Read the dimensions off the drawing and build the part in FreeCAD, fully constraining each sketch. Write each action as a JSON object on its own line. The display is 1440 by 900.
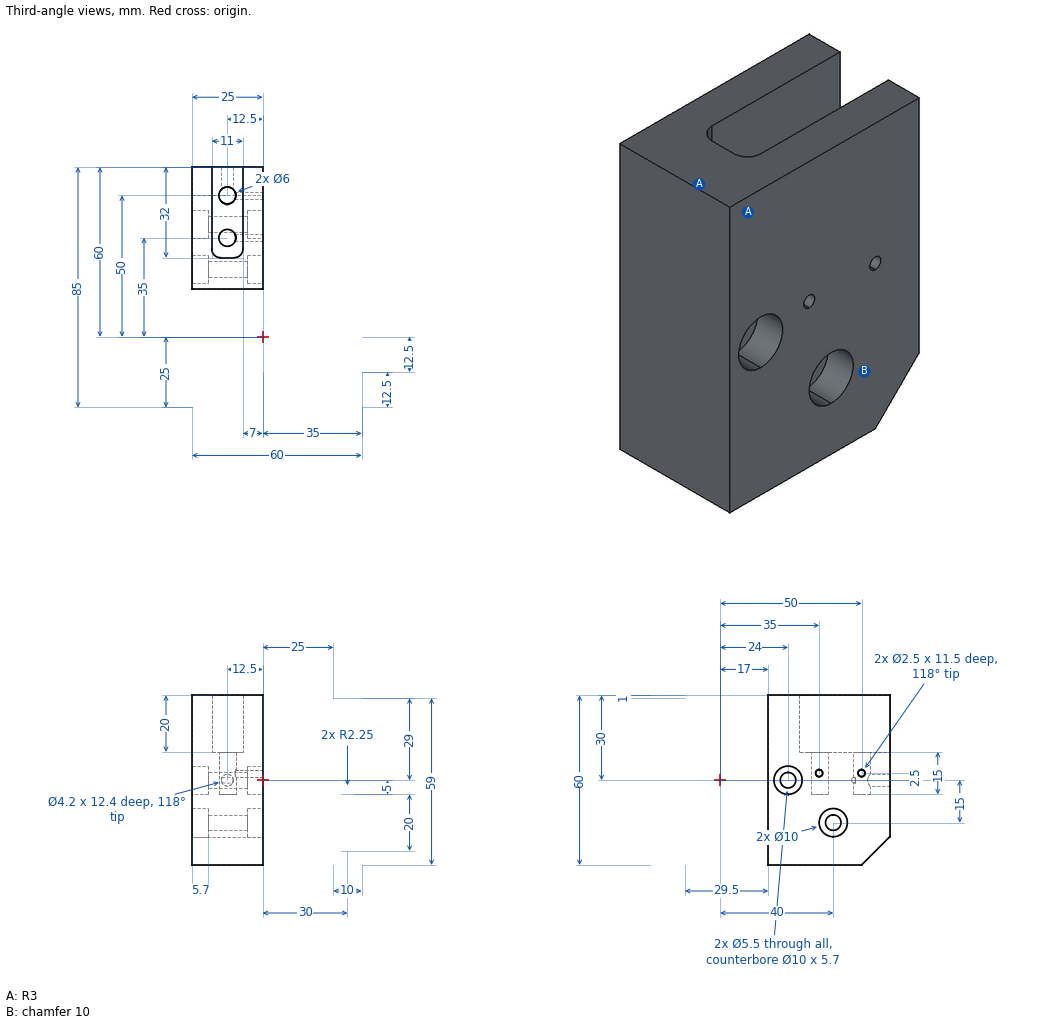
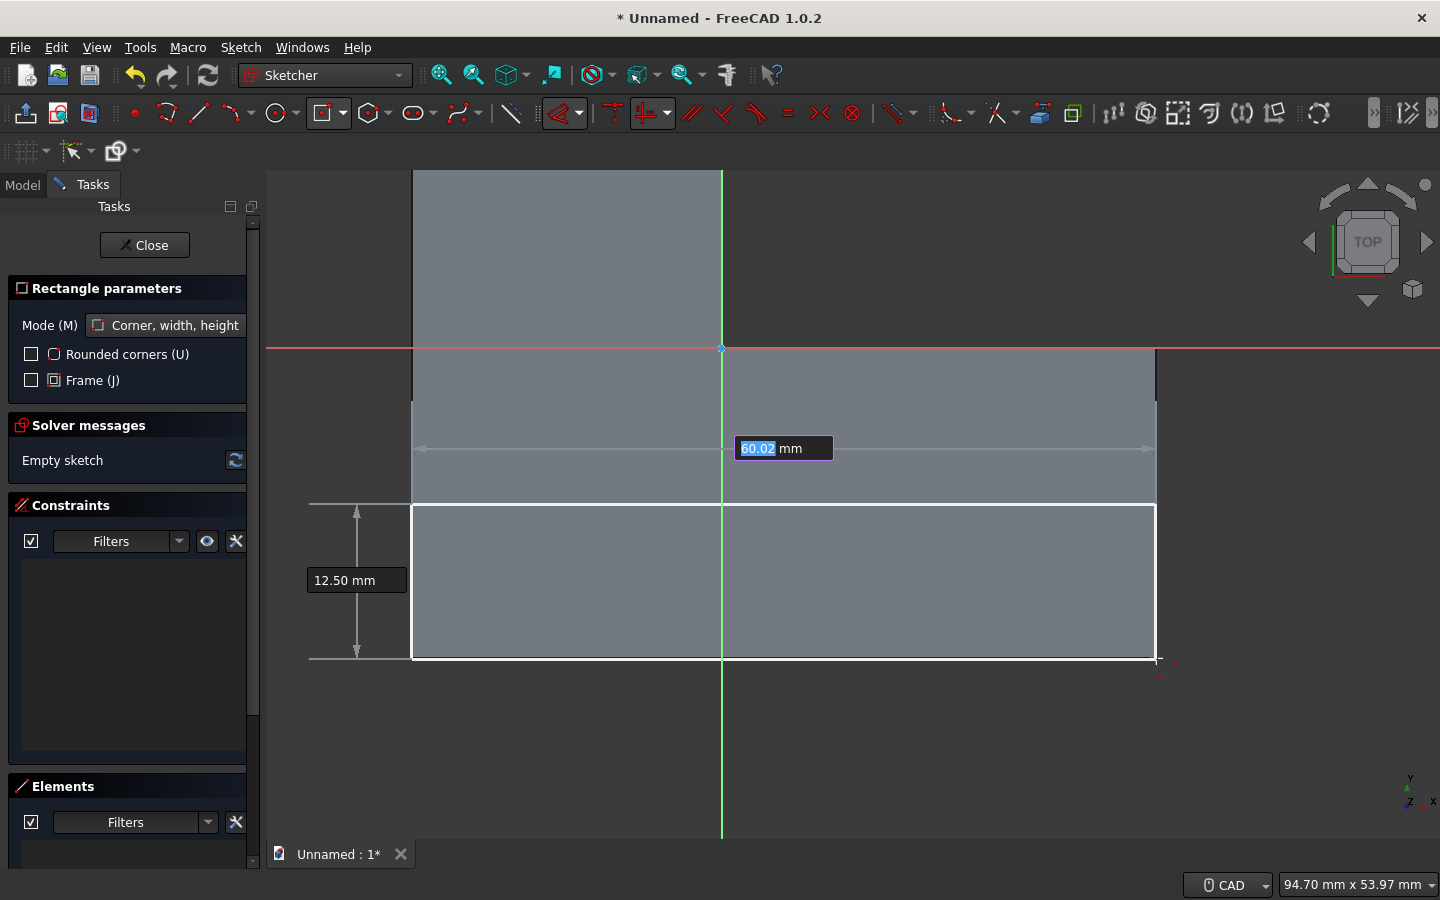
{"action": "type", "text": "60"}
{"action": "key", "text": "Tab"}
{"action": "type", "text": "12.5"}
{"action": "key", "text": "Return"}
{"action": "key", "text": "Escape"}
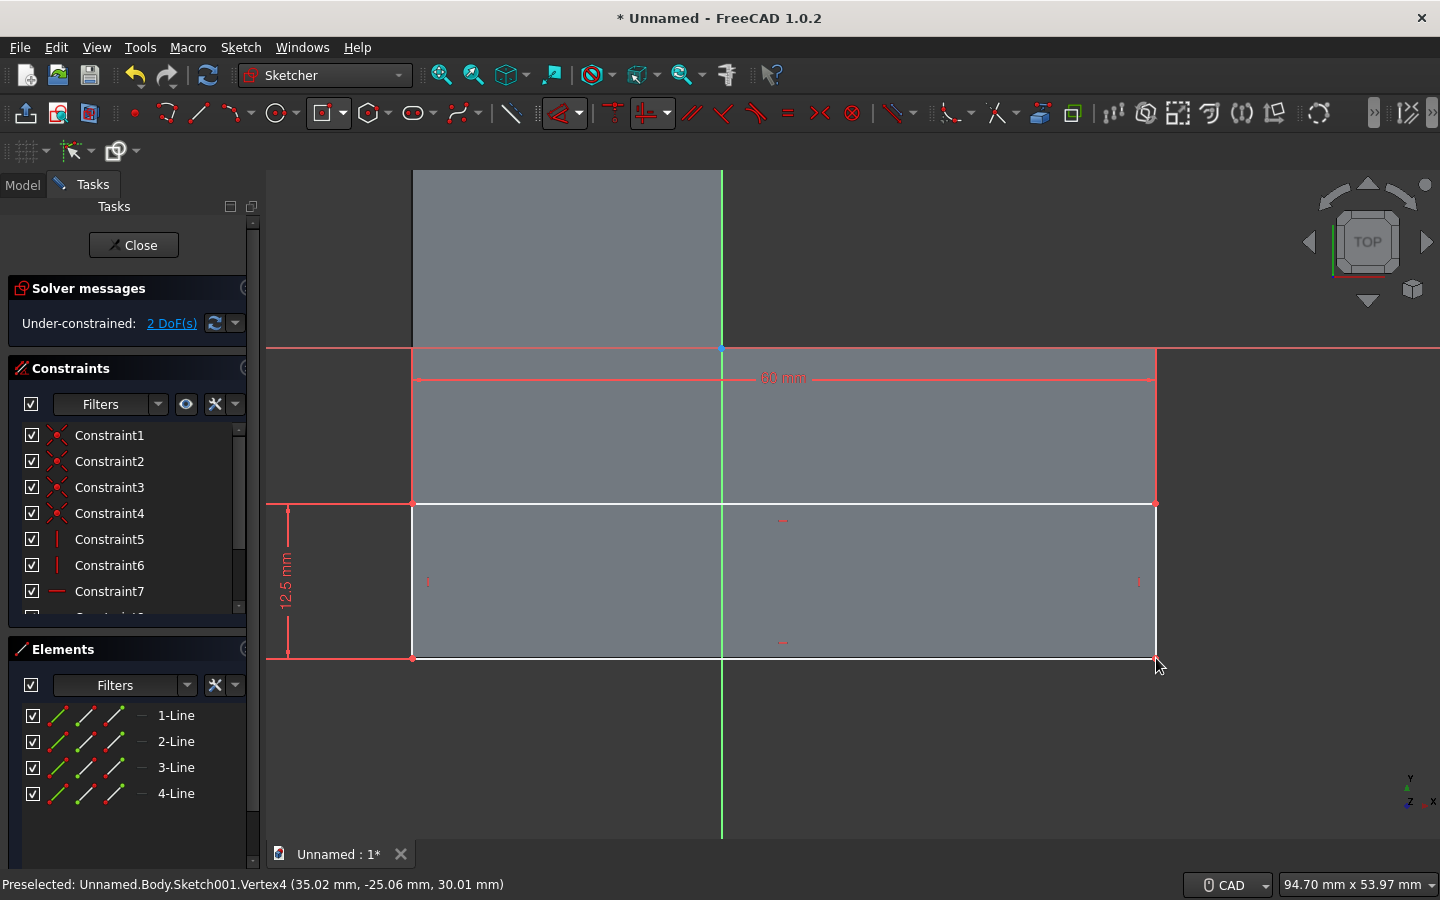
{"action": "left_click", "coordinate": [412, 504]}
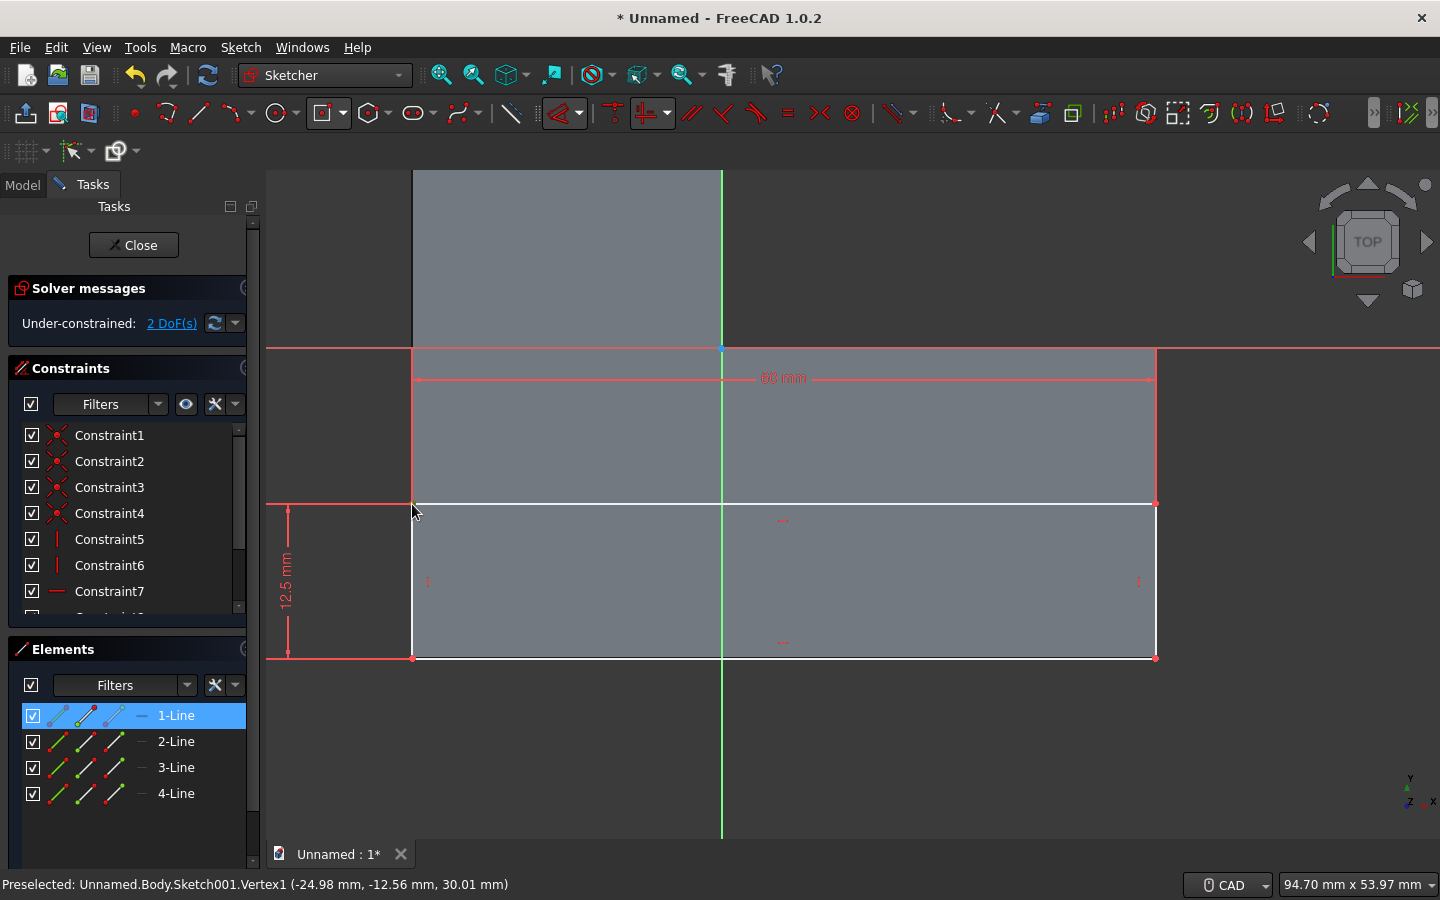
{"action": "left_click", "coordinate": [582, 114]}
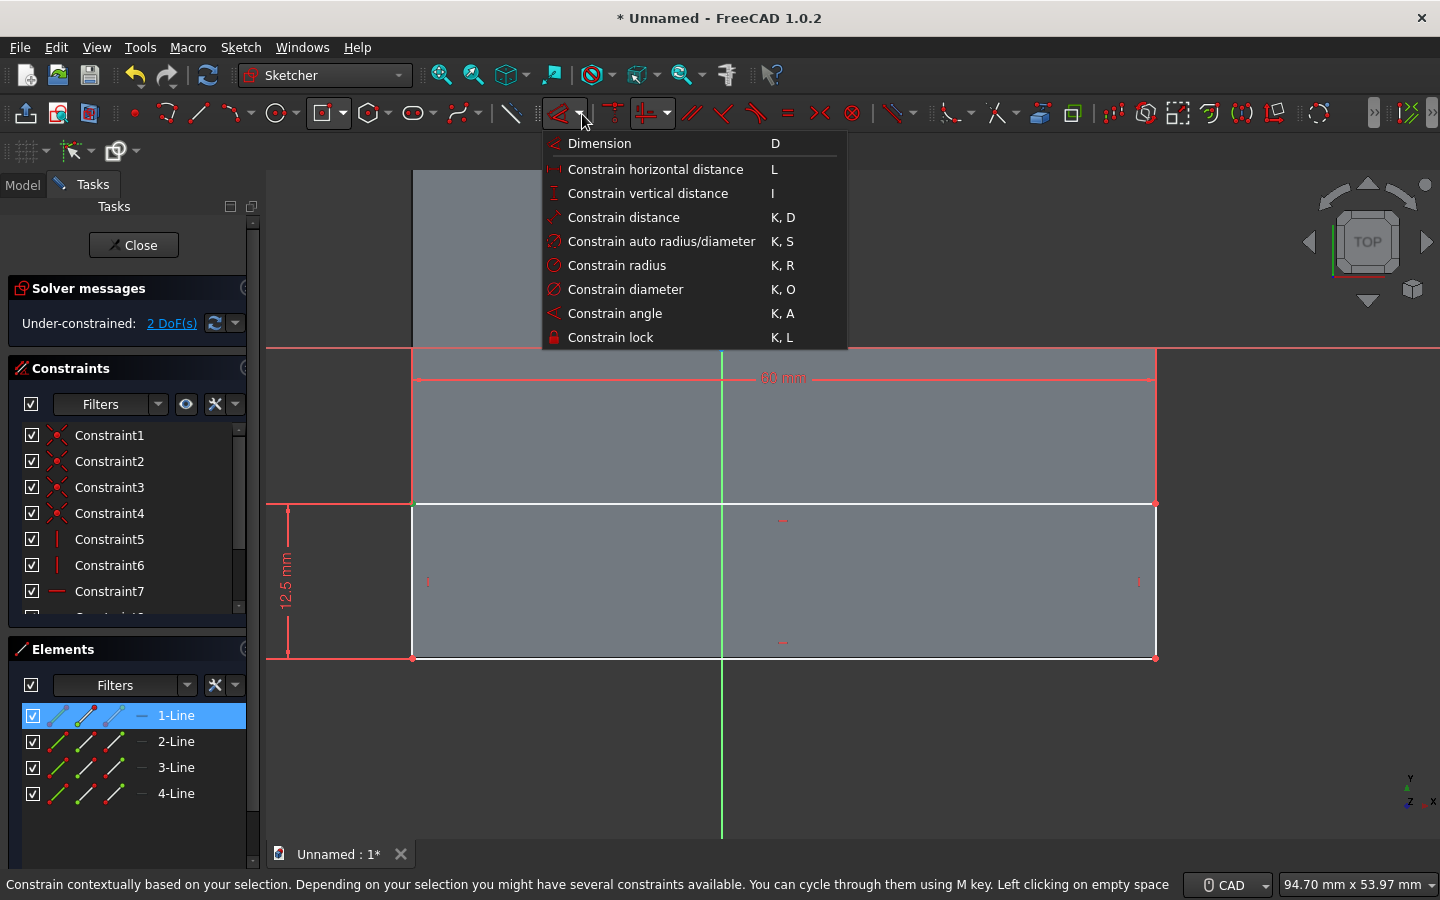
{"action": "left_click", "coordinate": [695, 169]}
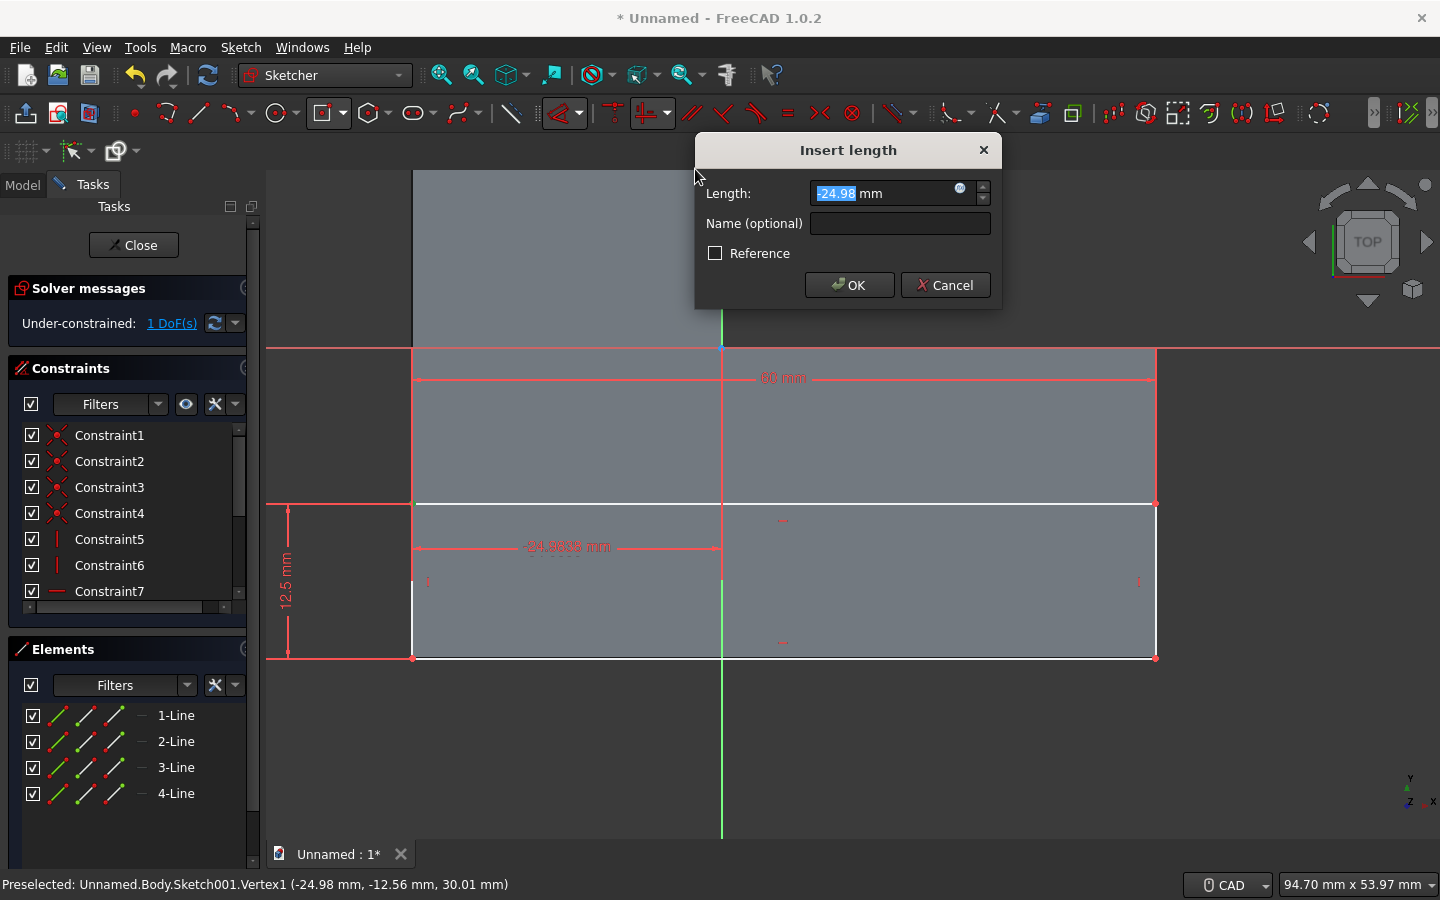
{"action": "type", "text": "-25"}
{"action": "key", "text": "Return"}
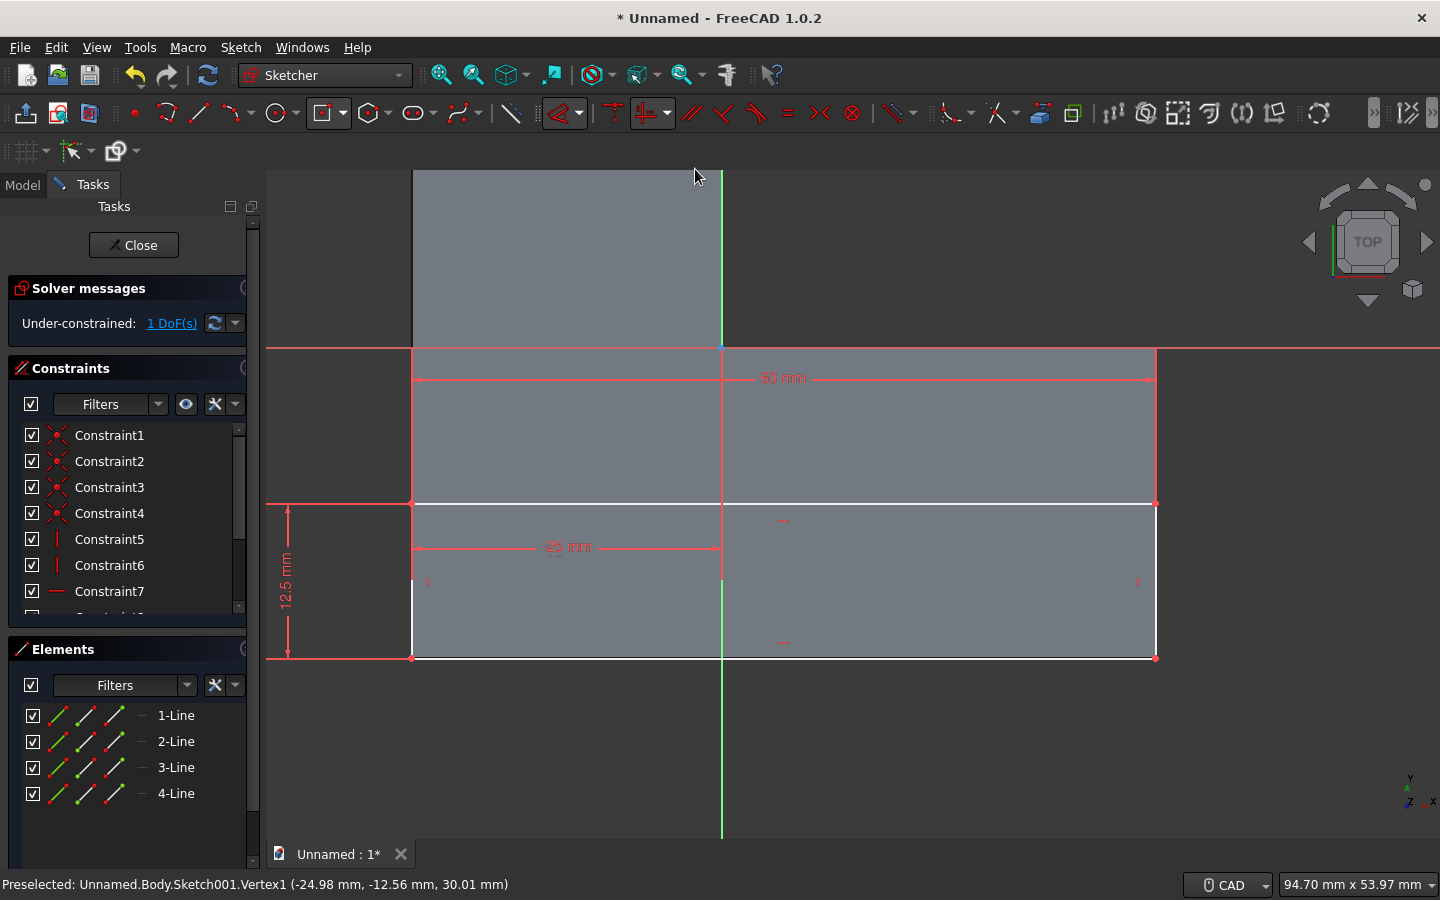
{"action": "left_click", "coordinate": [412, 659]}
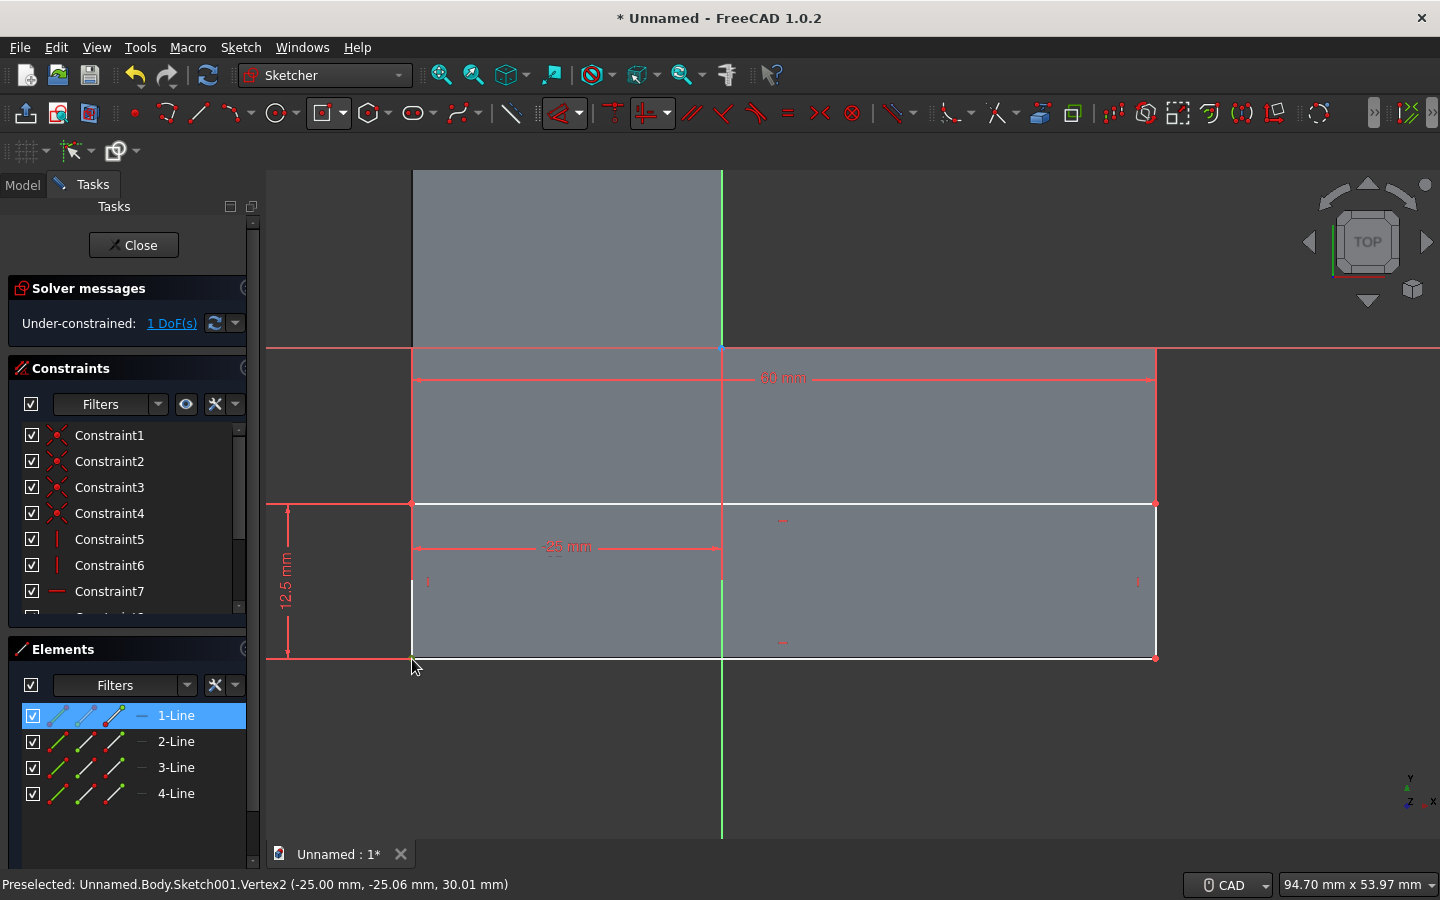
{"action": "key", "text": "i"}